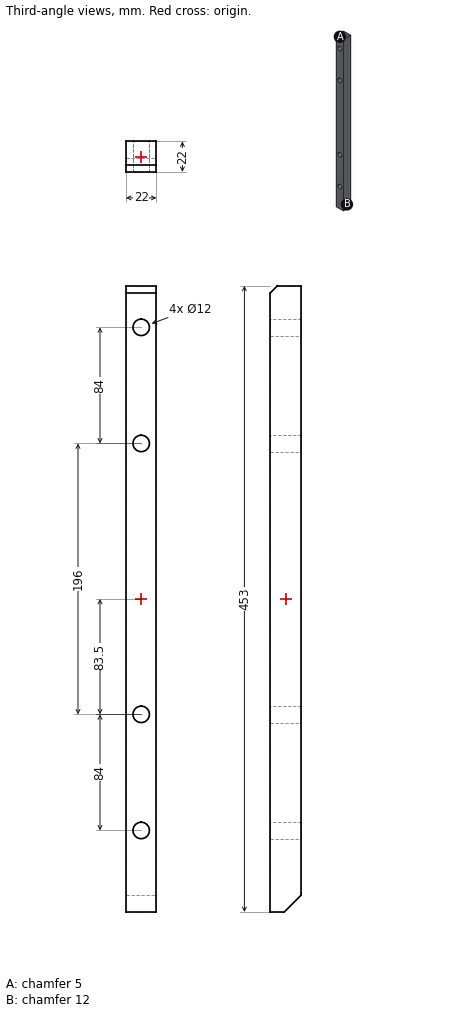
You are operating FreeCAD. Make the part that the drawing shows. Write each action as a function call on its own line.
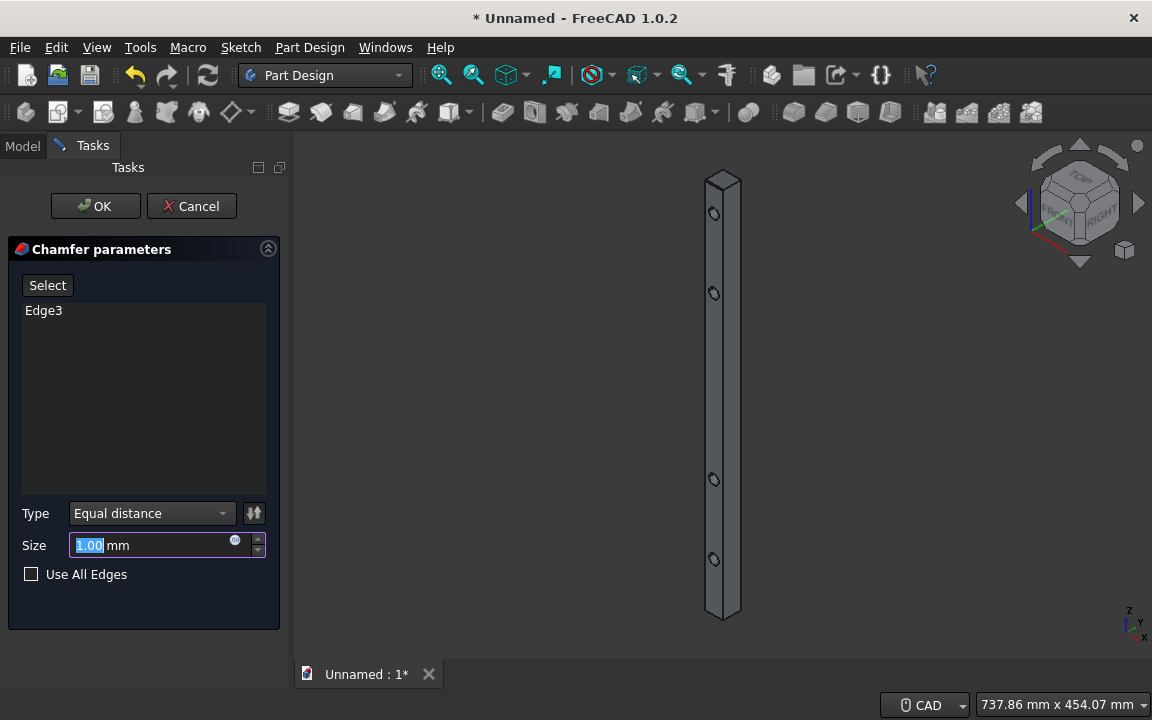
text(5)
key(Tab)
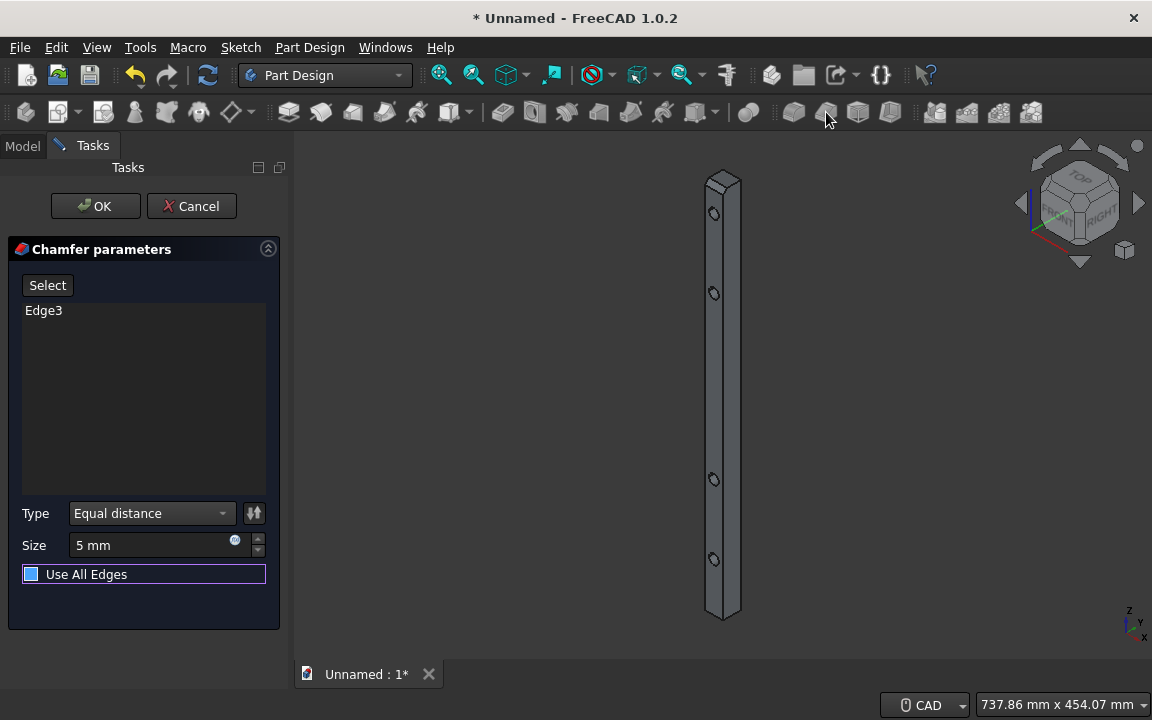
click(96, 206)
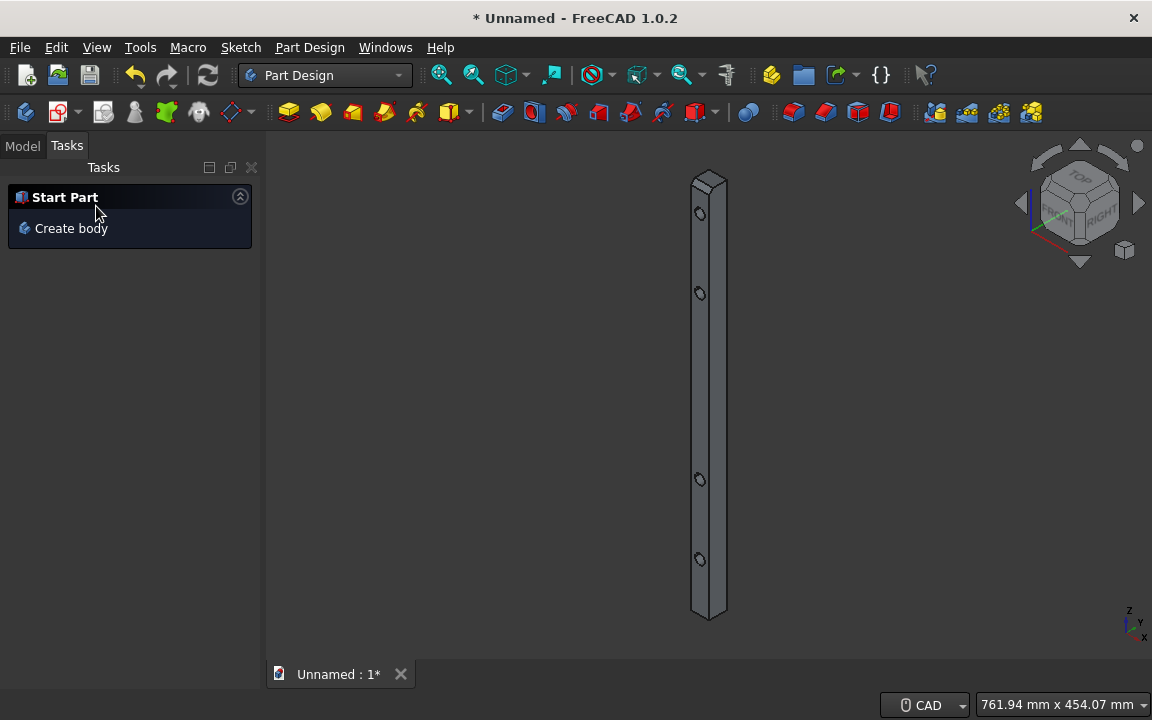
key(2)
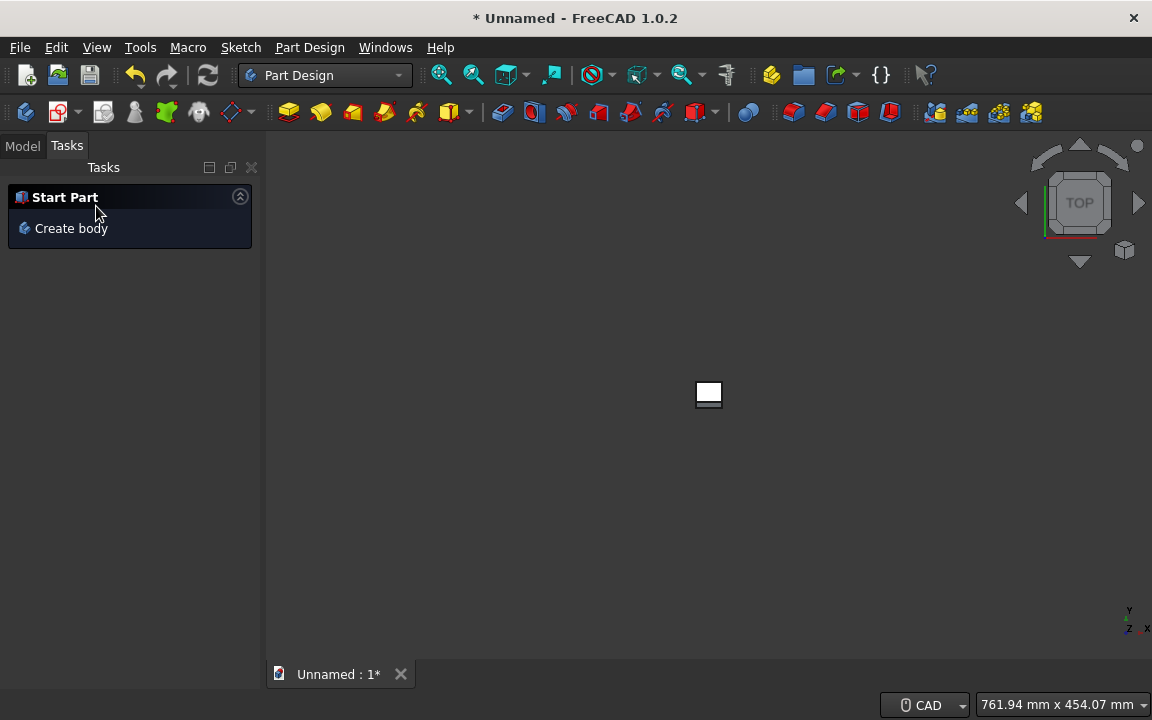
key(v)
key(f)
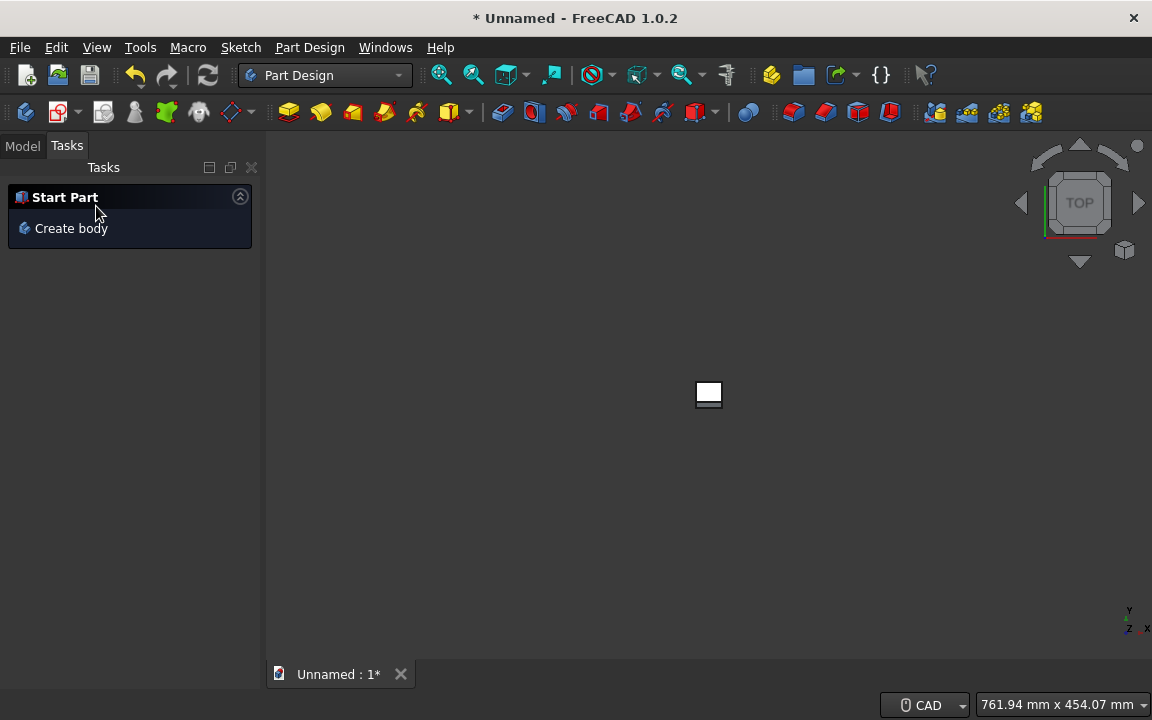
key(0)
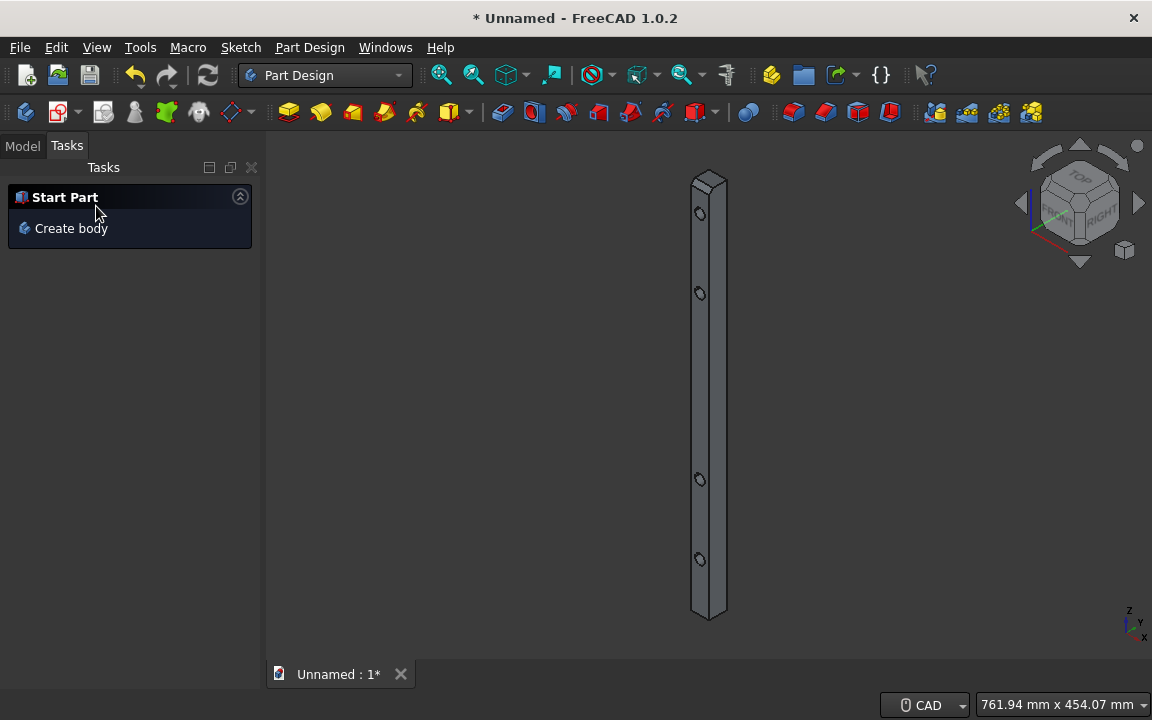
key(1)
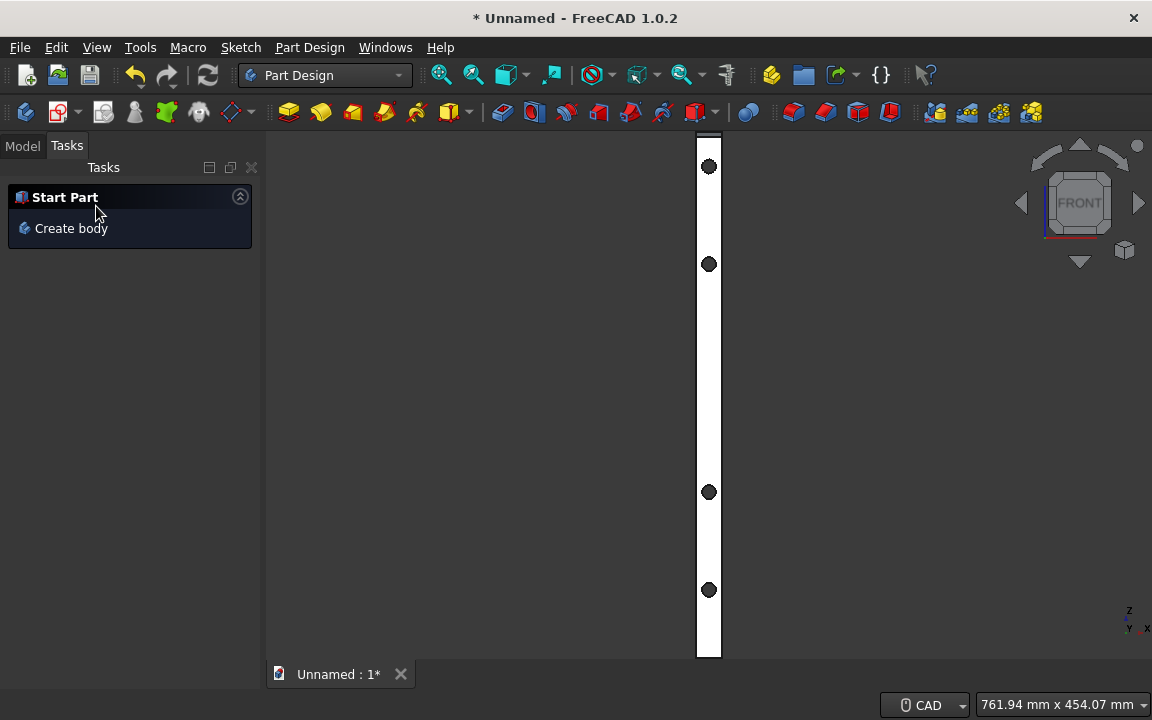
key(3)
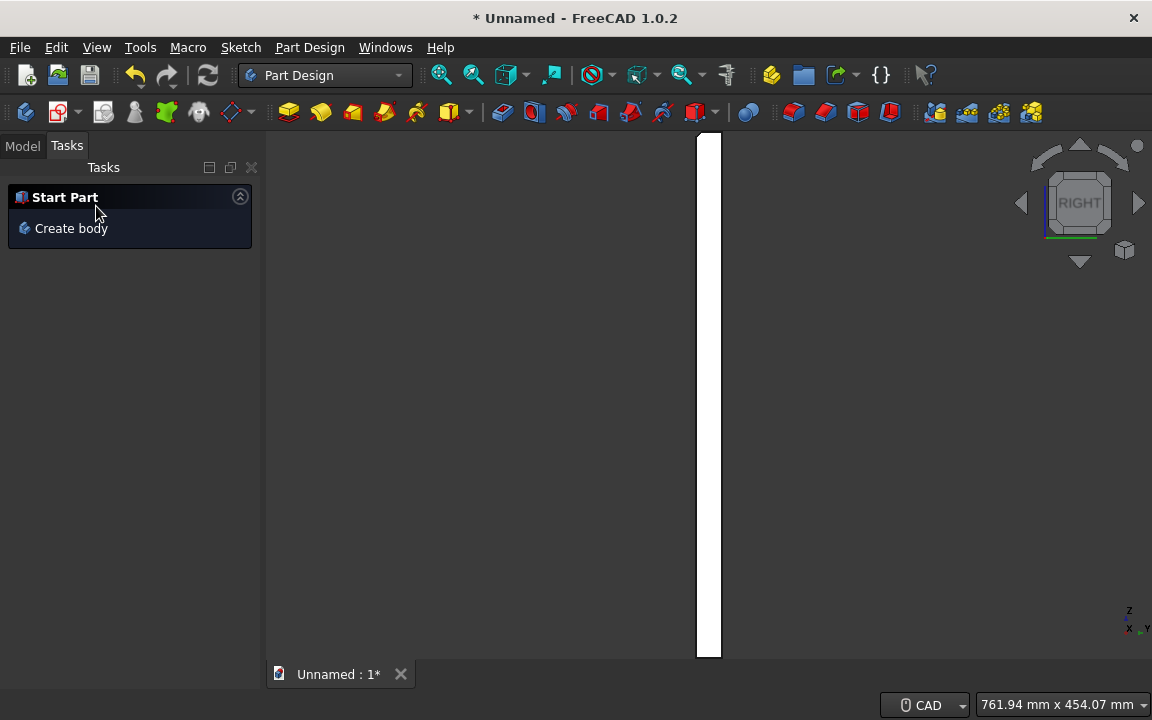
key(5)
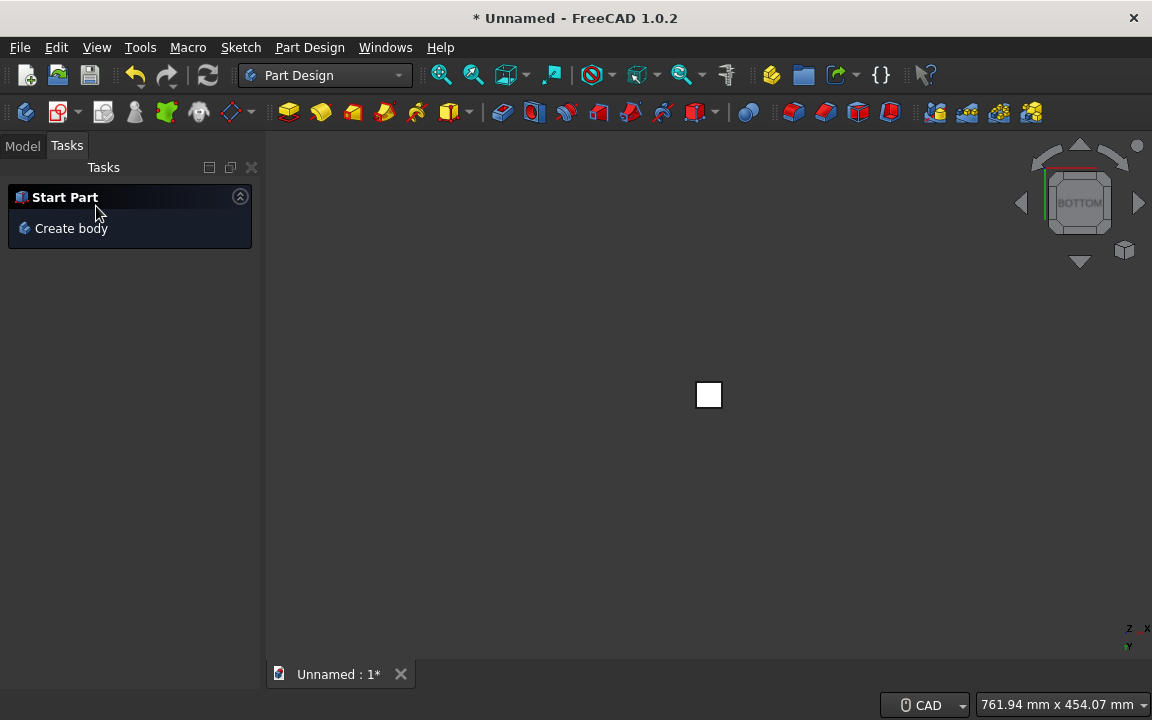
click(442, 76)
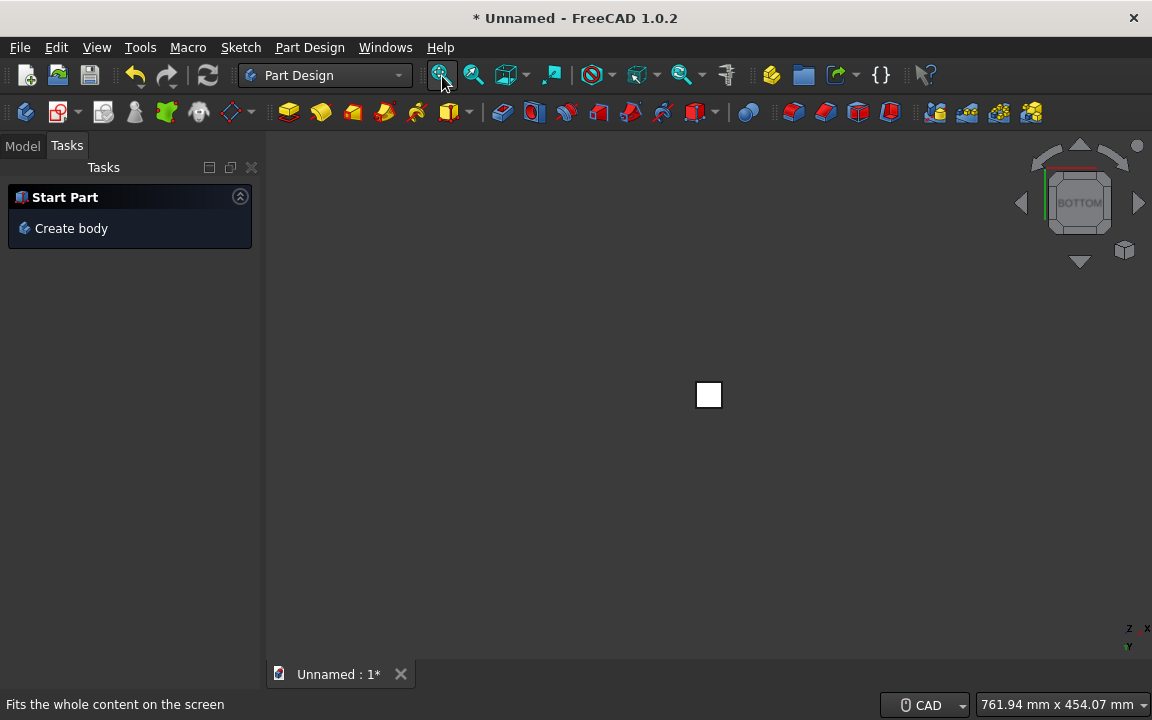
click(709, 407)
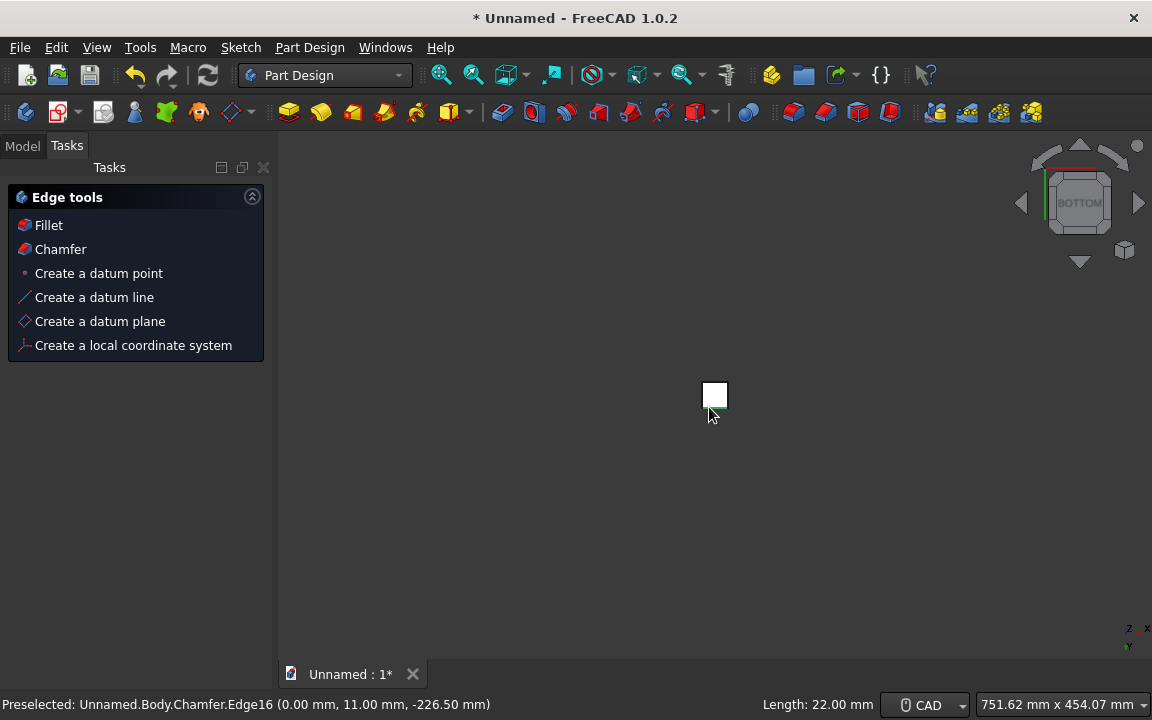
click(826, 112)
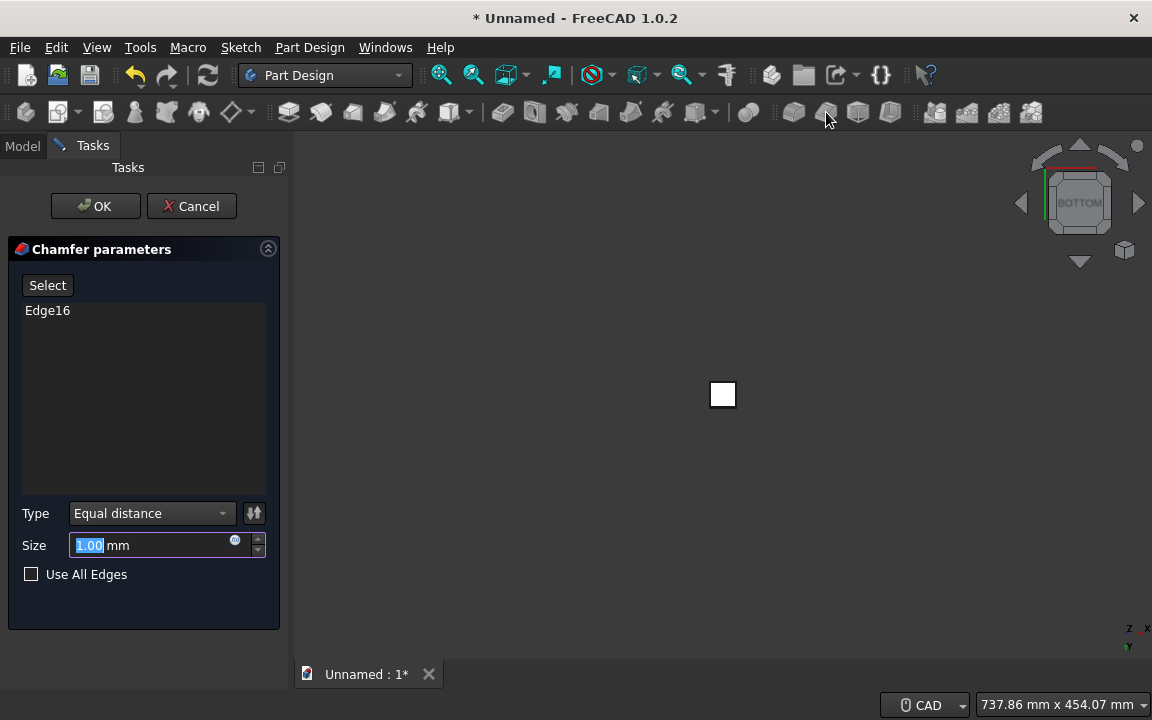
text(12)
key(Tab)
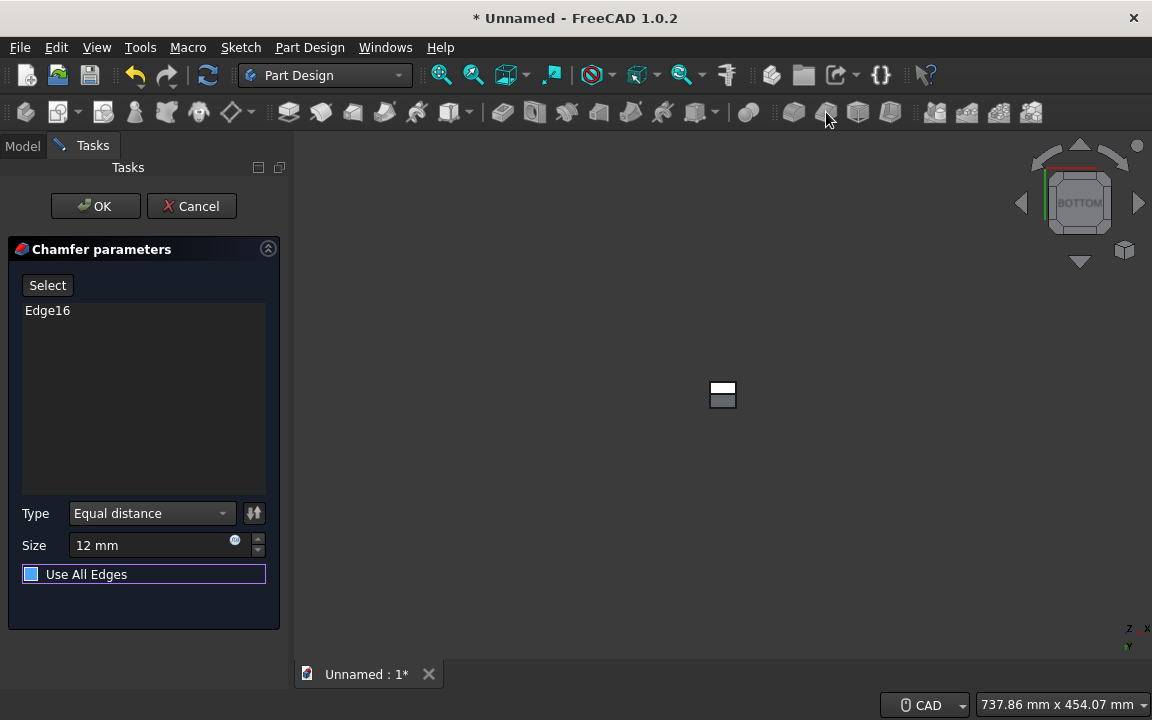
click(96, 206)